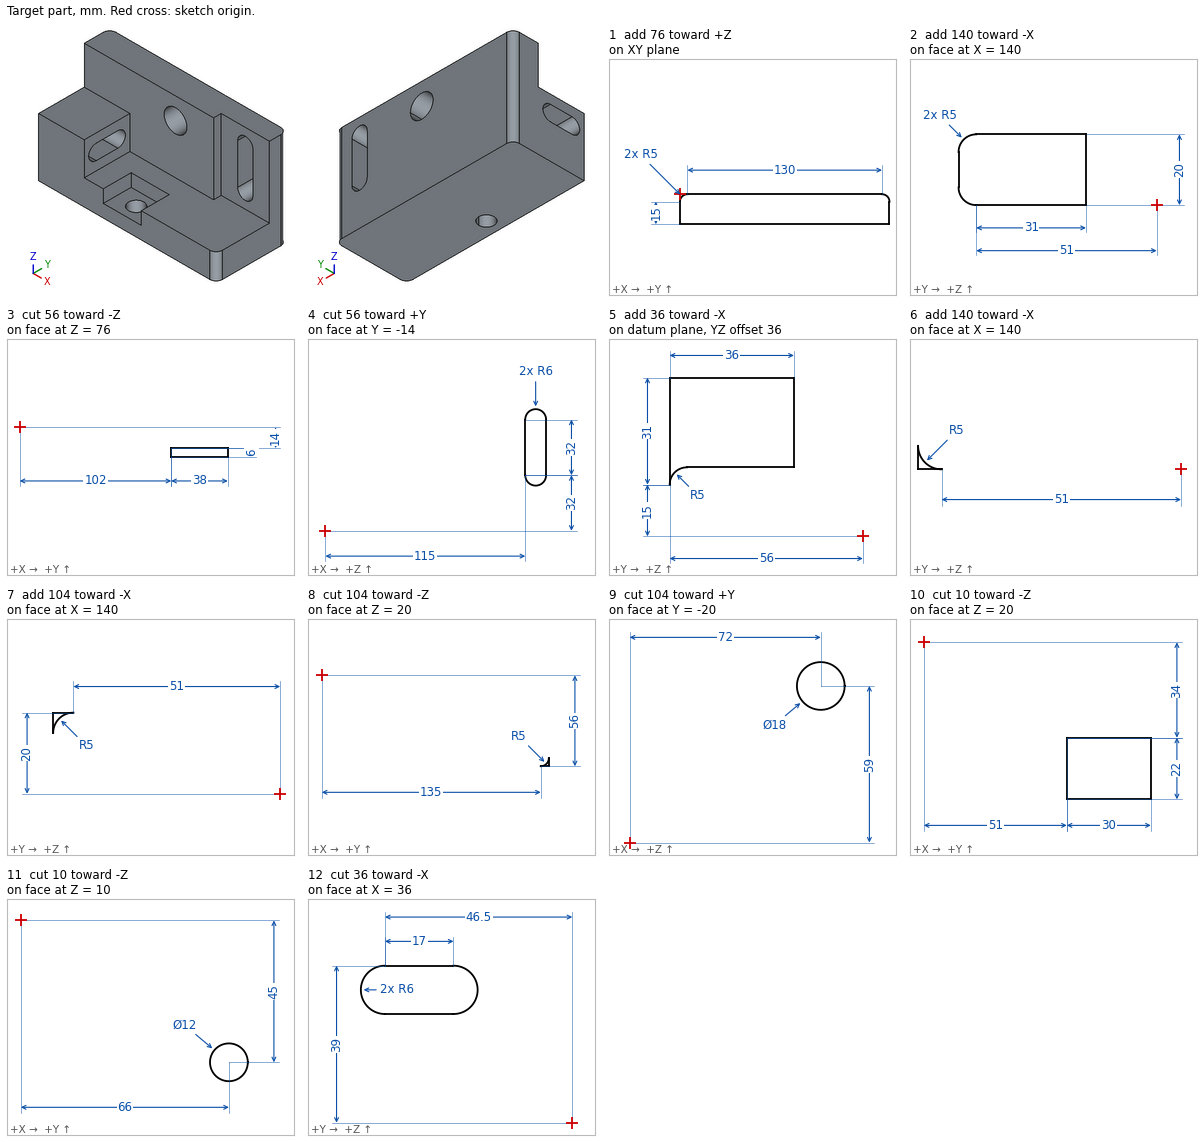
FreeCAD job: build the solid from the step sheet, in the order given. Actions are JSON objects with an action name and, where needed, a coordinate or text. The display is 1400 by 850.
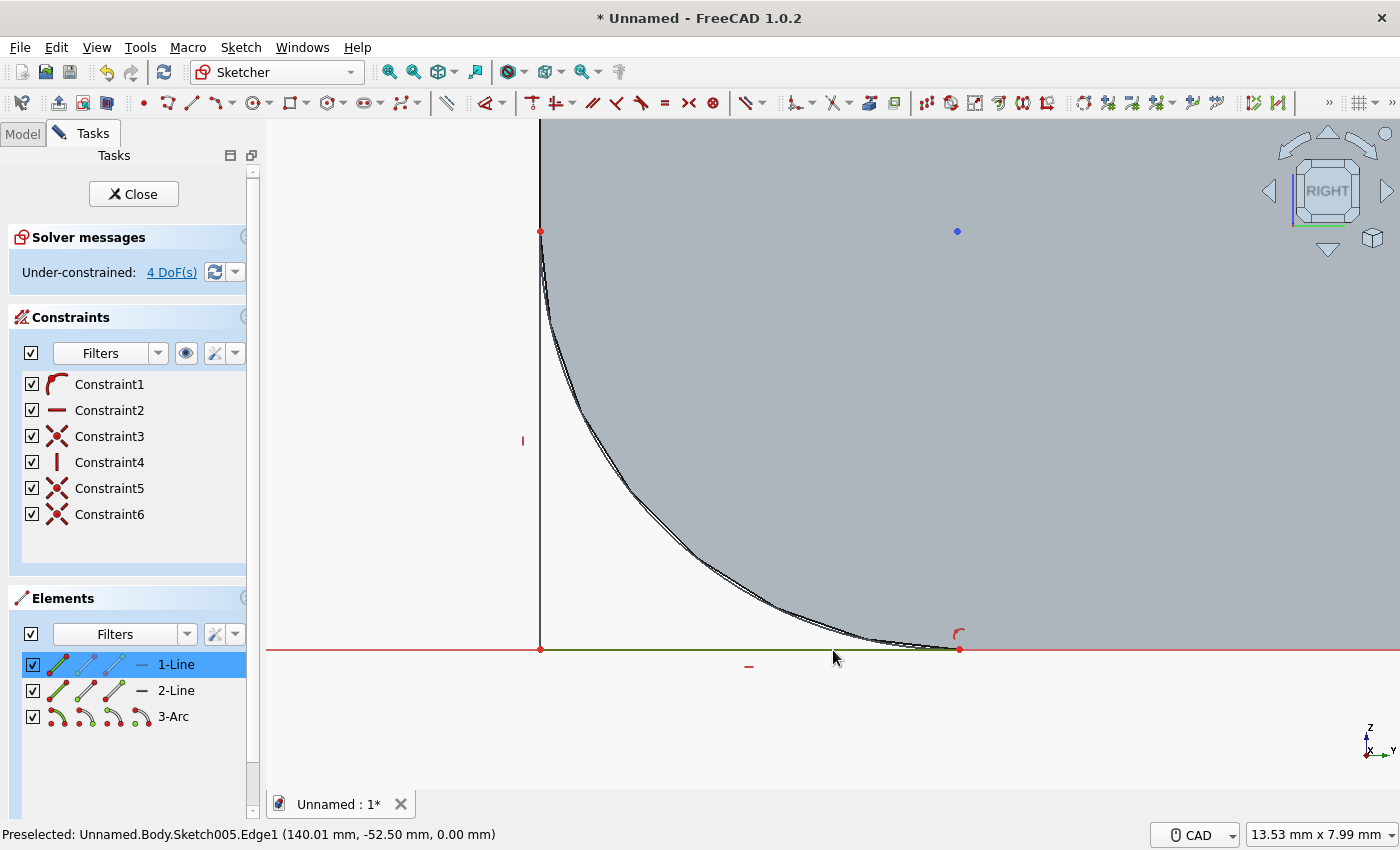
{"action": "left_click", "coordinate": [586, 422]}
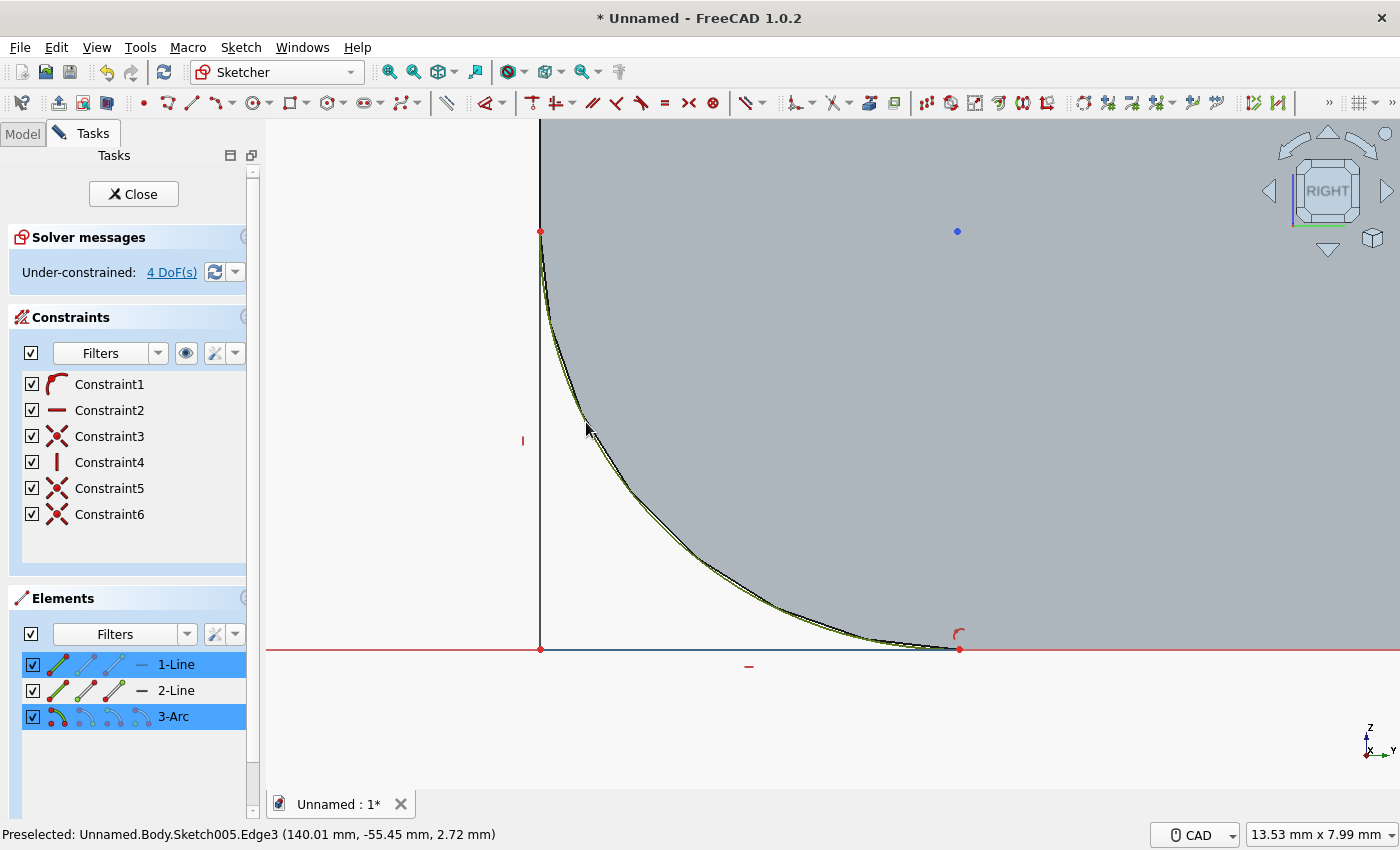
{"action": "key", "text": "t"}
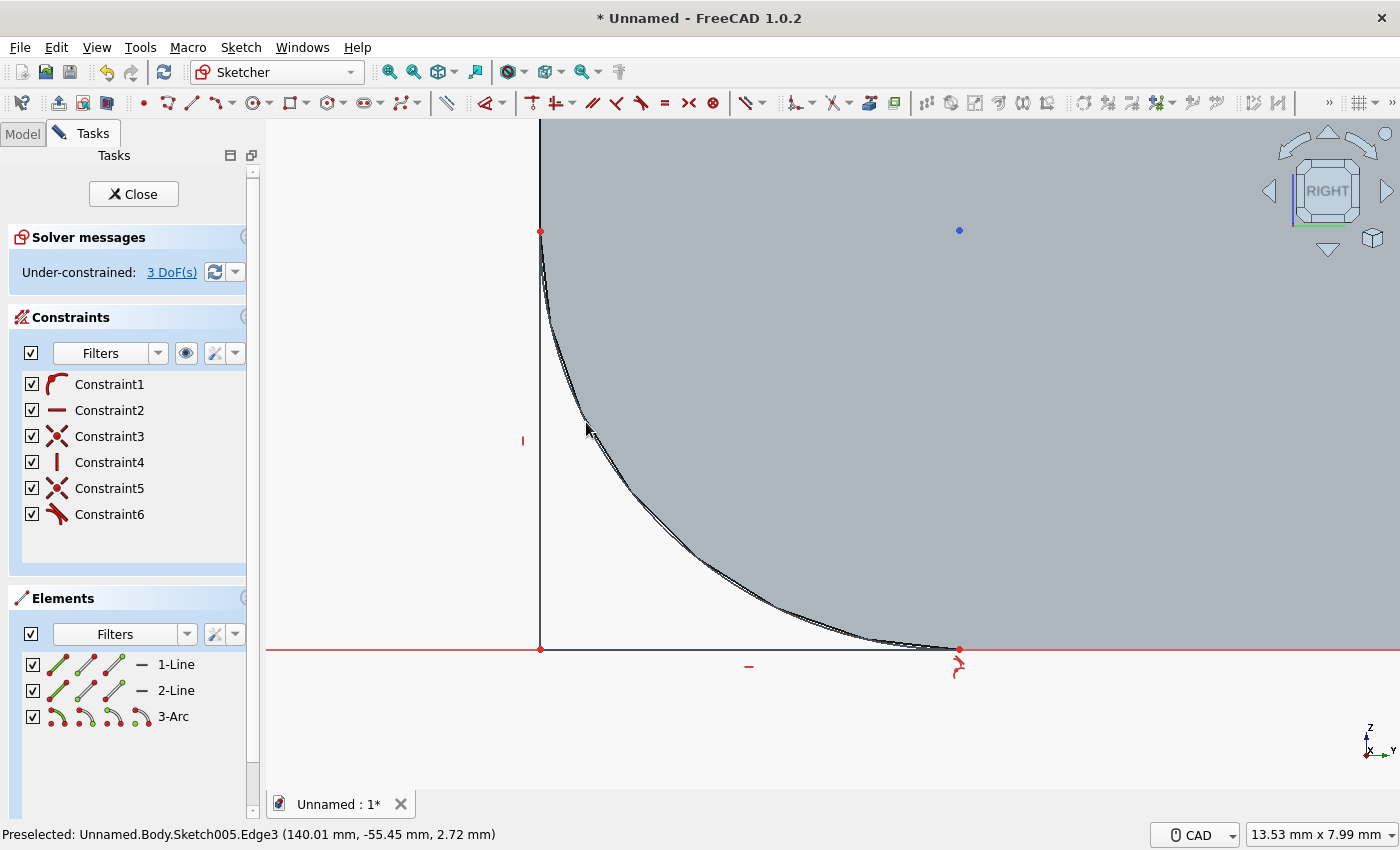
{"action": "left_click", "coordinate": [540, 524]}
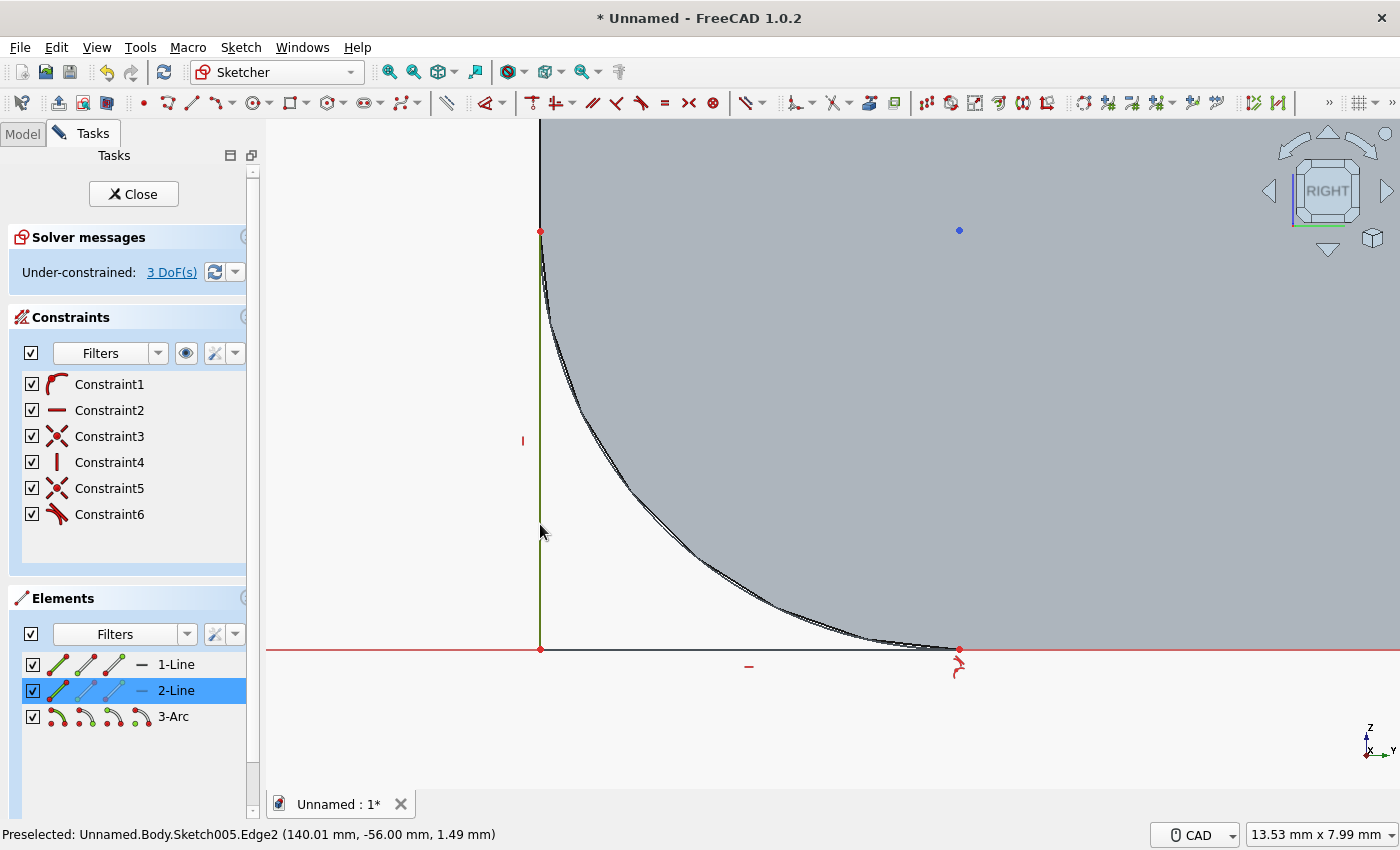
{"action": "left_click", "coordinate": [586, 422]}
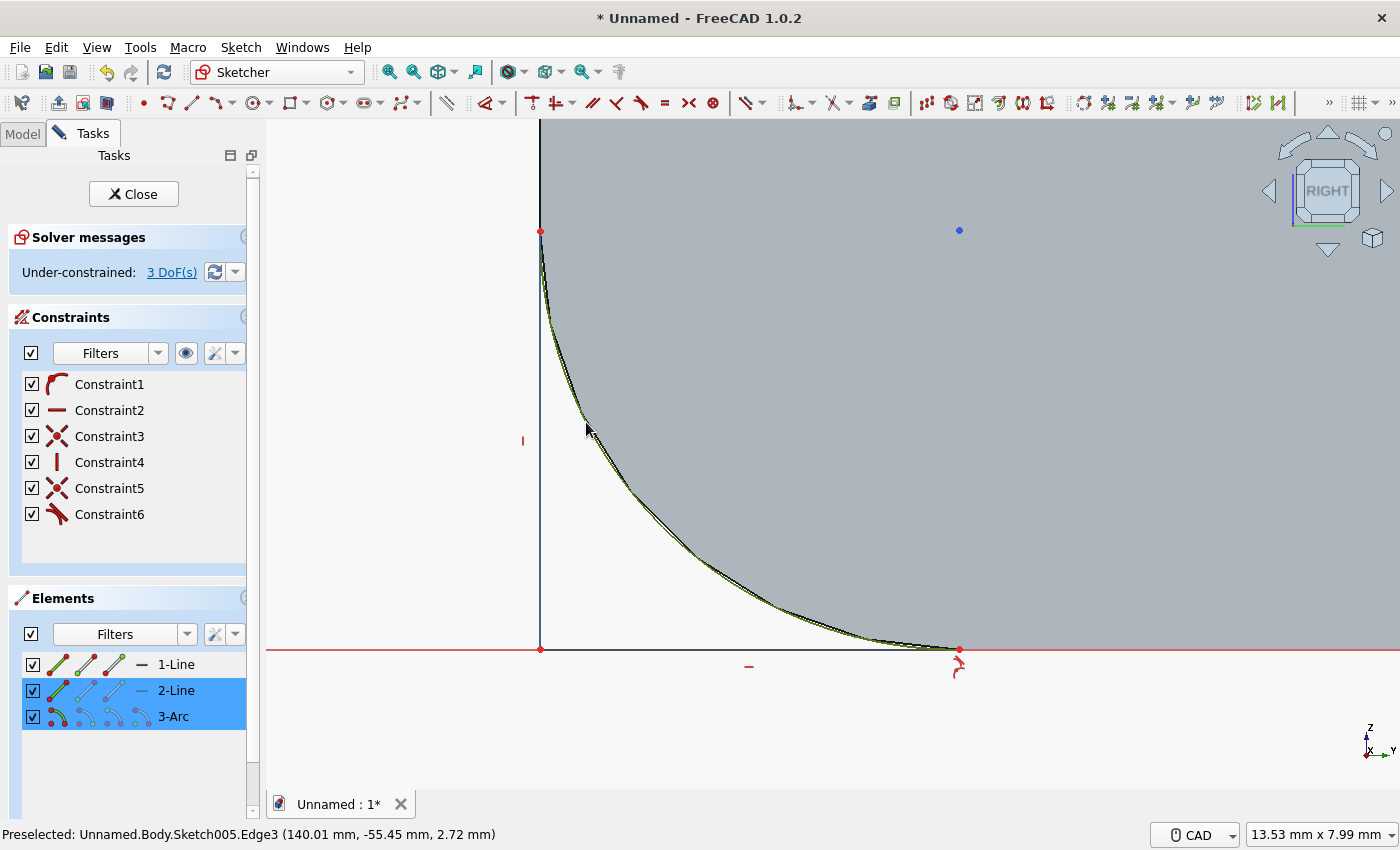
{"action": "left_click", "coordinate": [642, 104]}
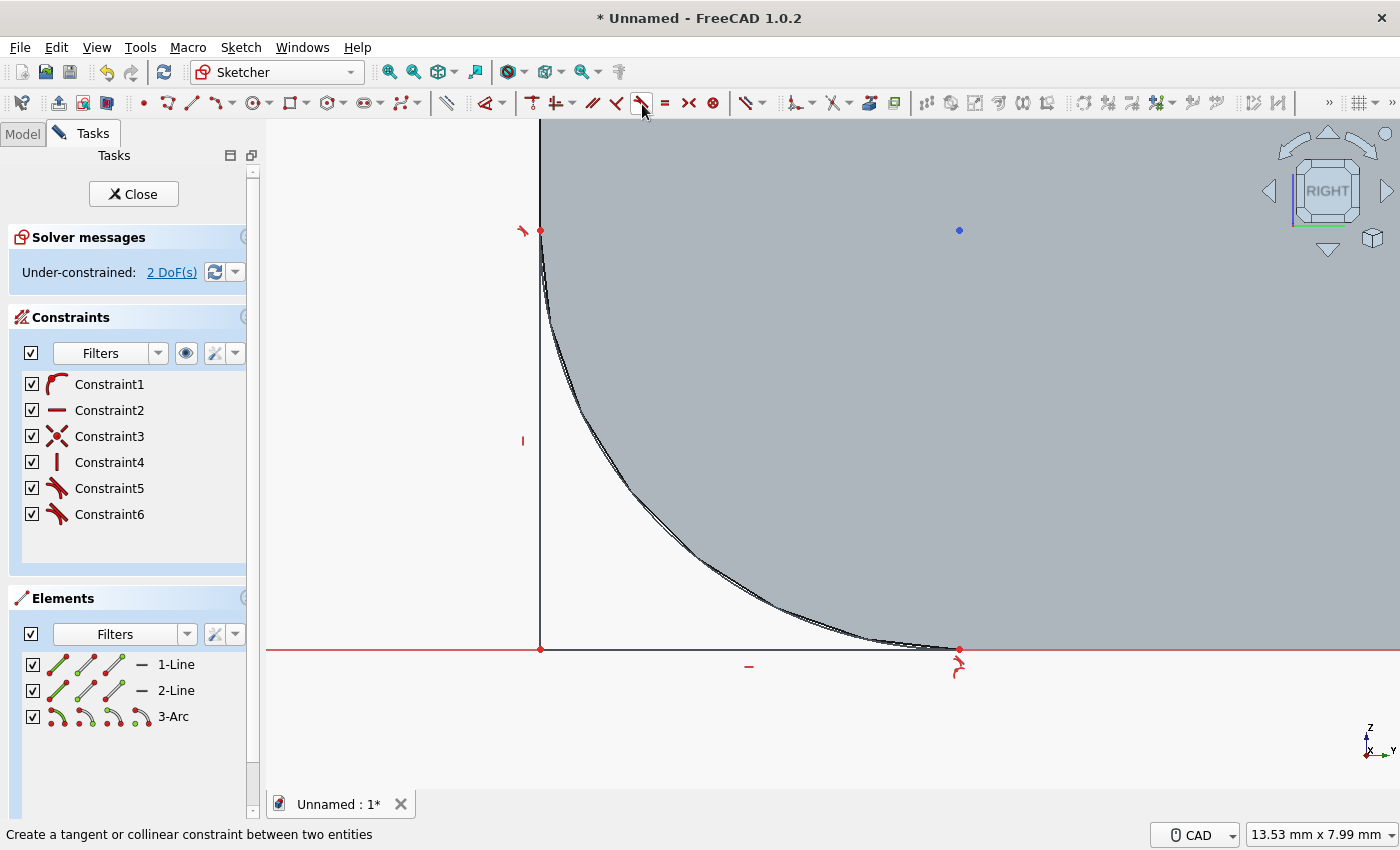
{"action": "left_click", "coordinate": [486, 104]}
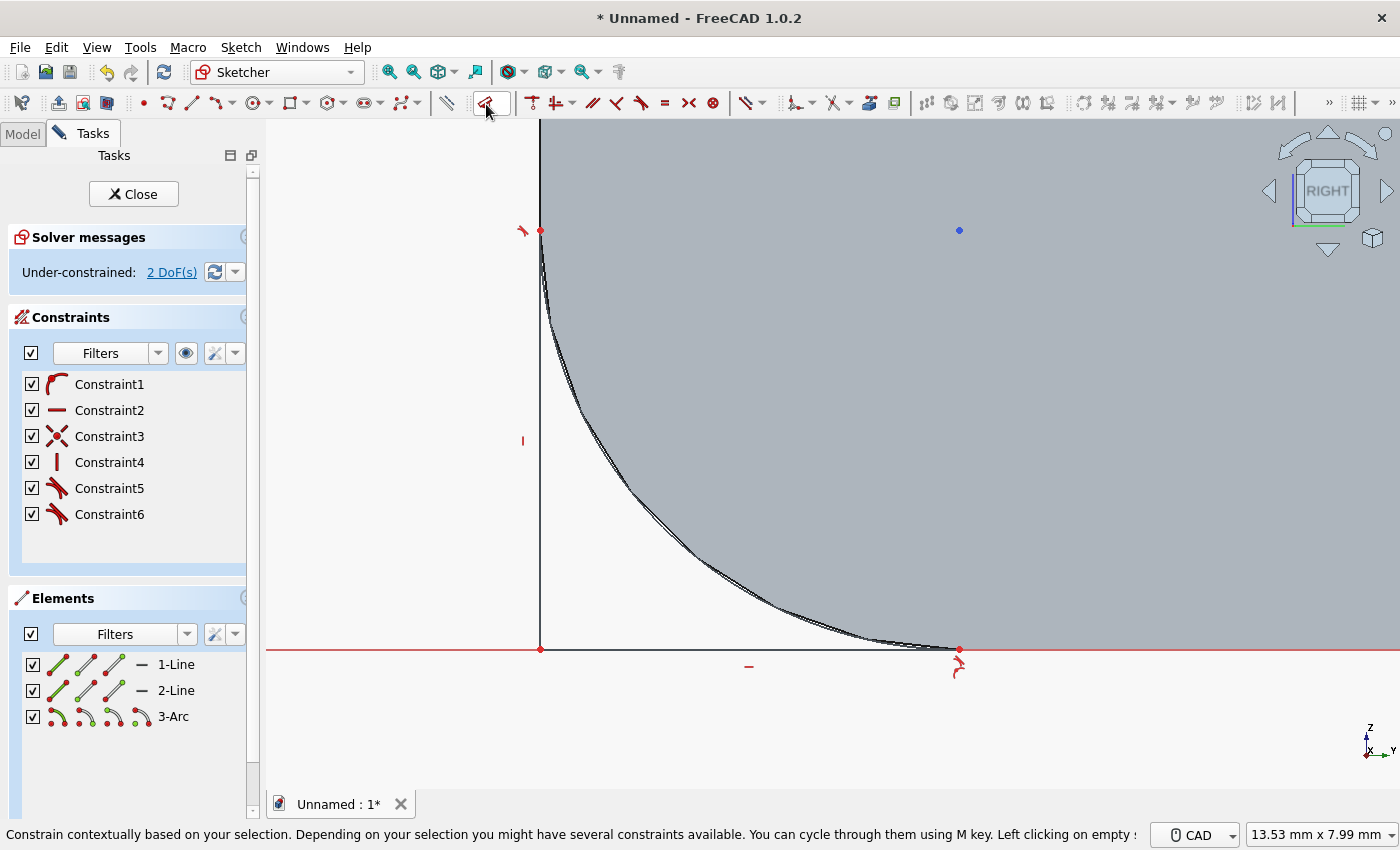
{"action": "left_click", "coordinate": [586, 421]}
{"action": "left_click", "coordinate": [557, 436]}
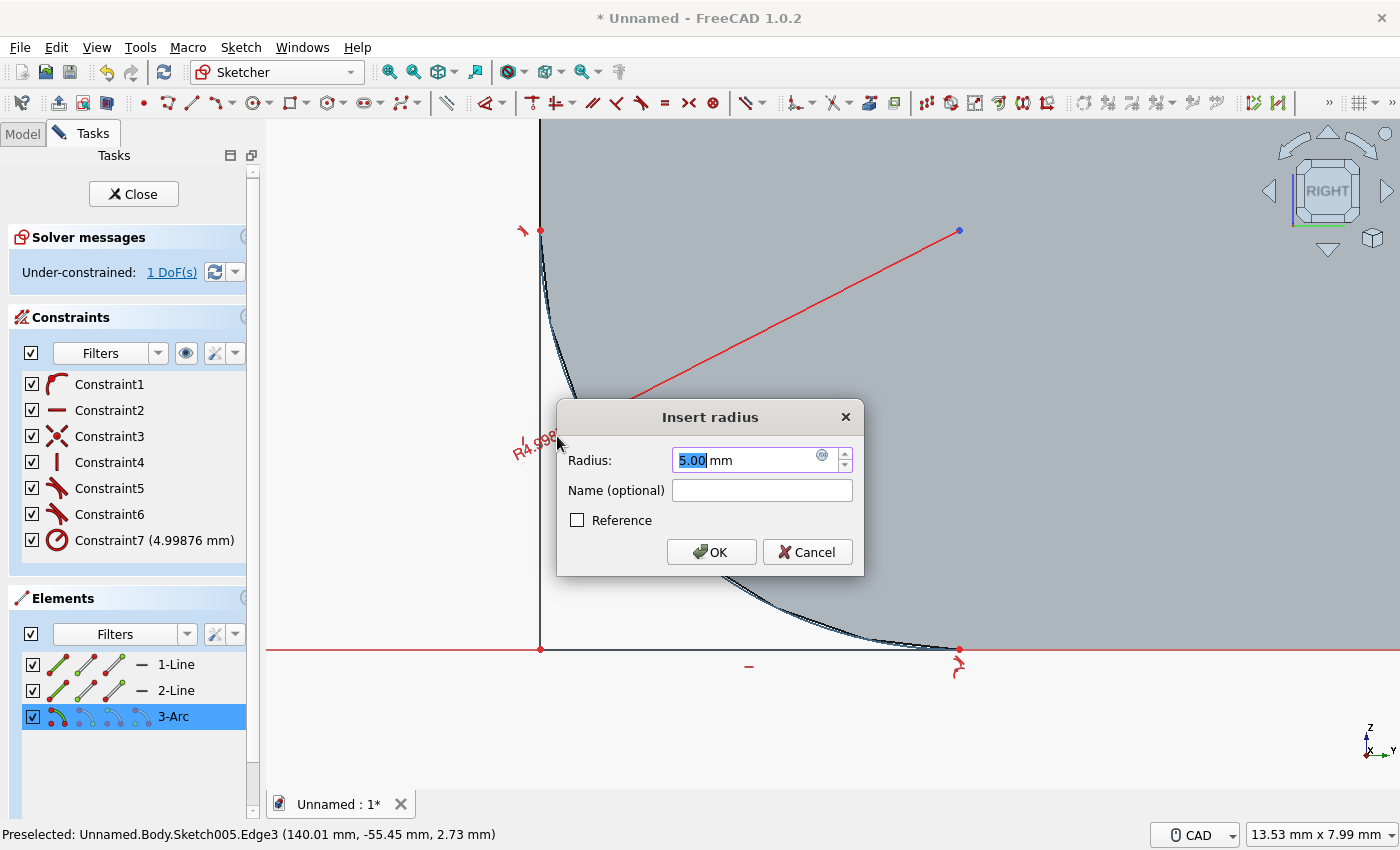
{"action": "type", "text": "5"}
{"action": "key", "text": "Return"}